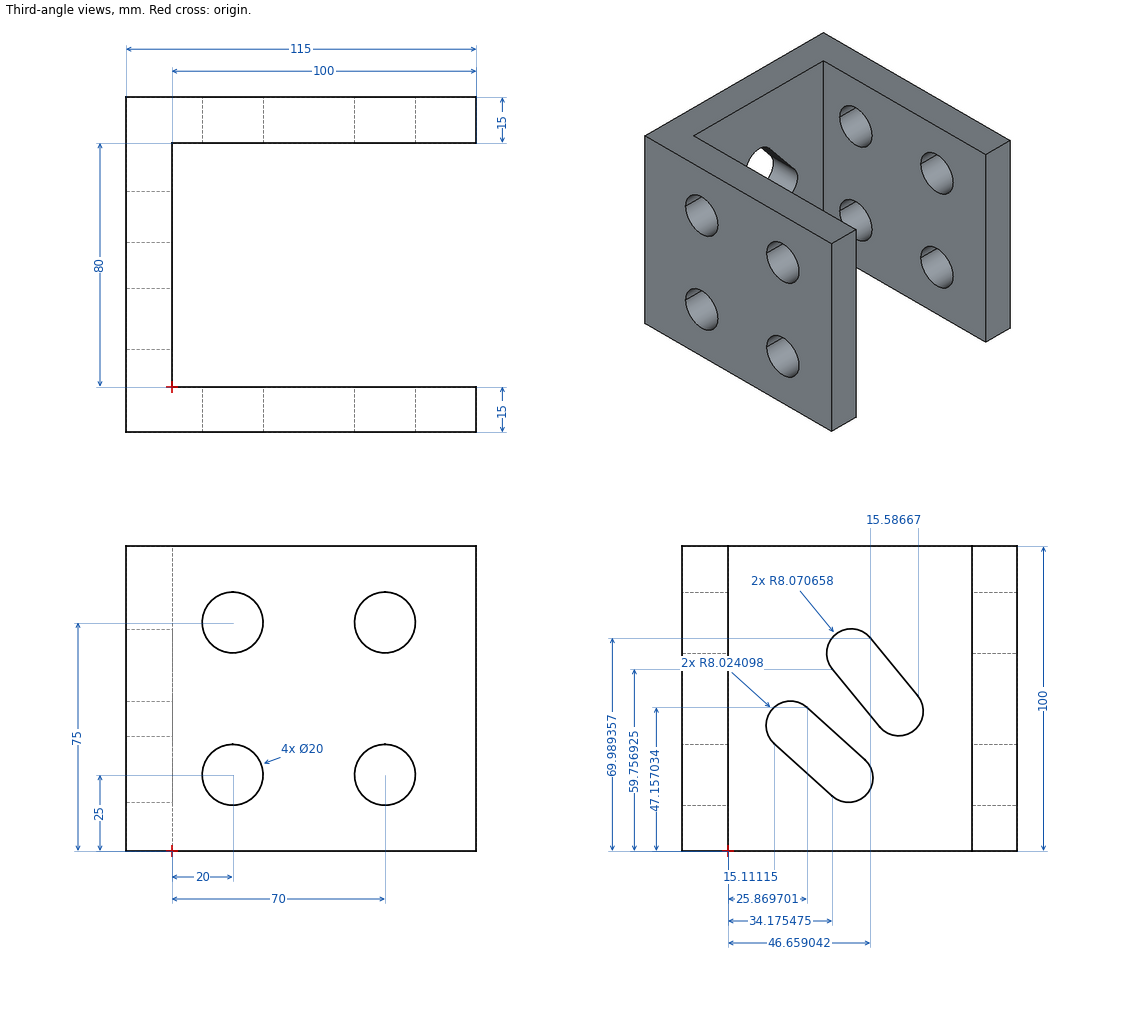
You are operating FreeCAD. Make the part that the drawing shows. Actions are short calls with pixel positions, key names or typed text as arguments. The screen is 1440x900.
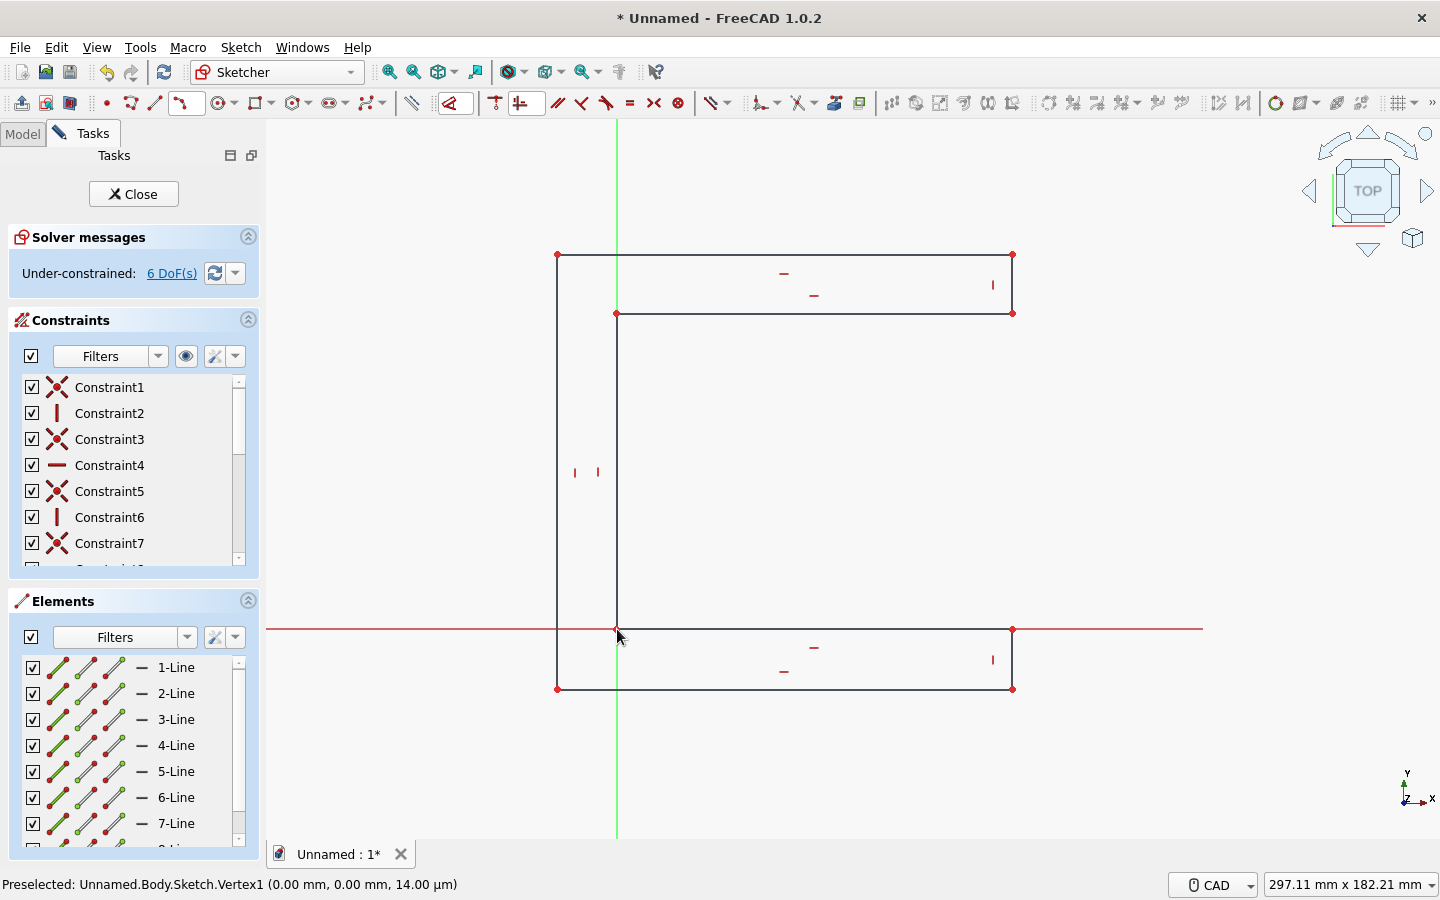
click(450, 104)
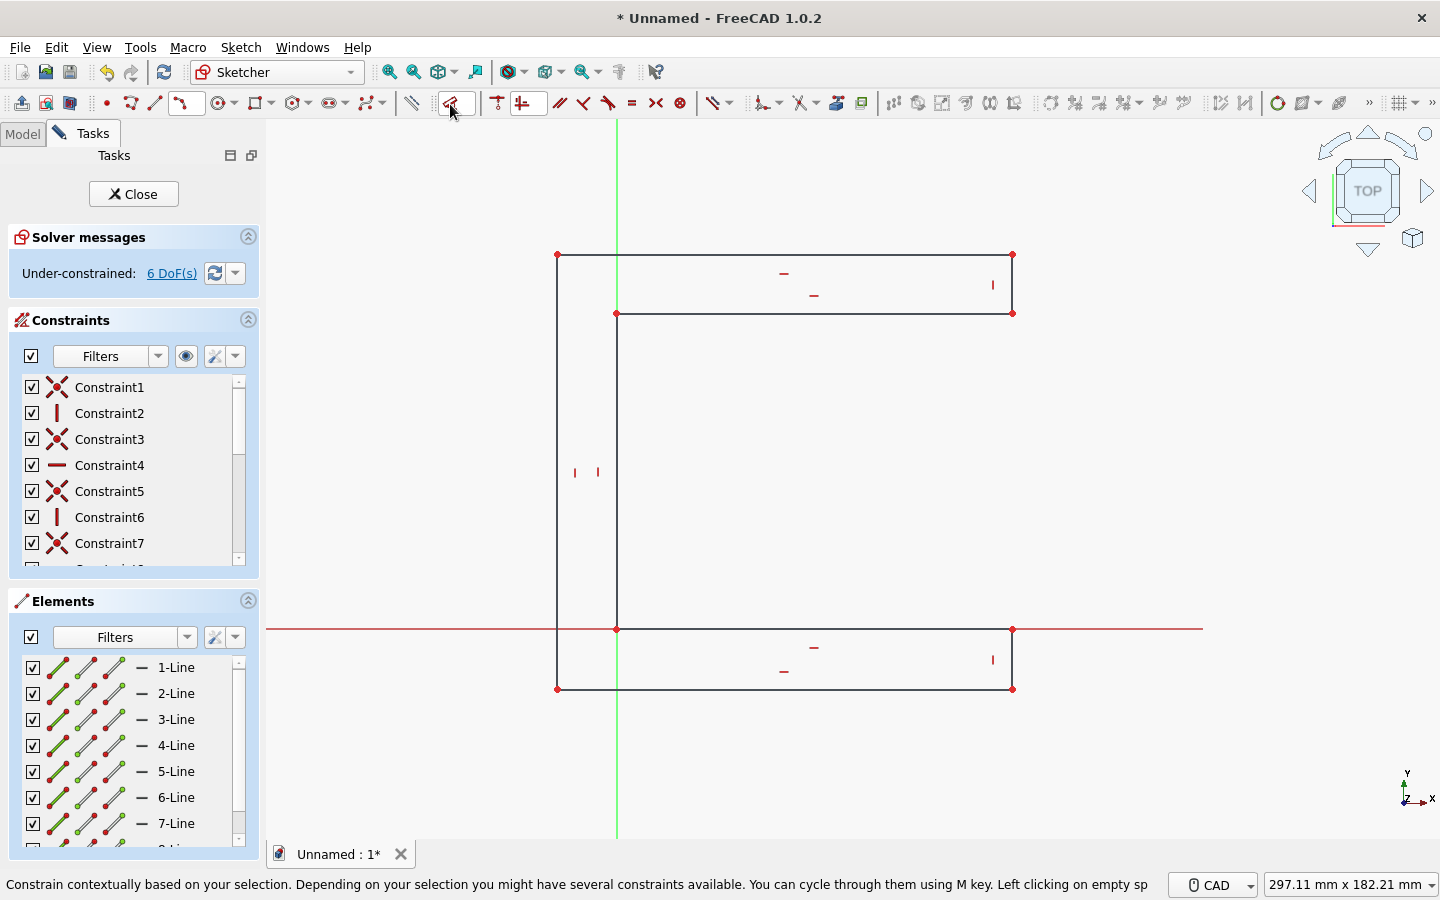
click(617, 535)
click(583, 472)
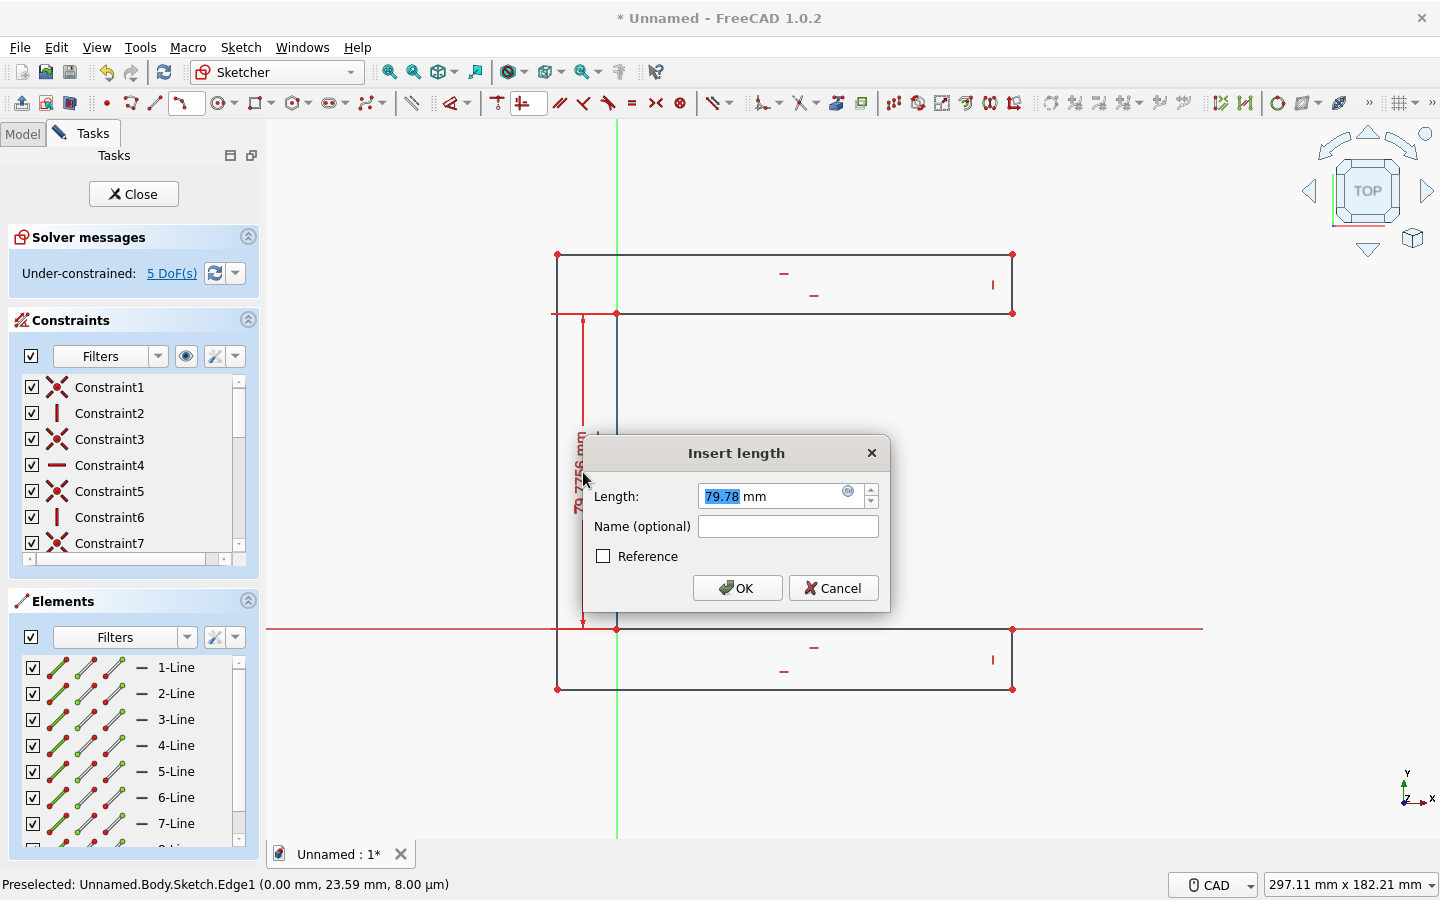
text(80)
key(Return)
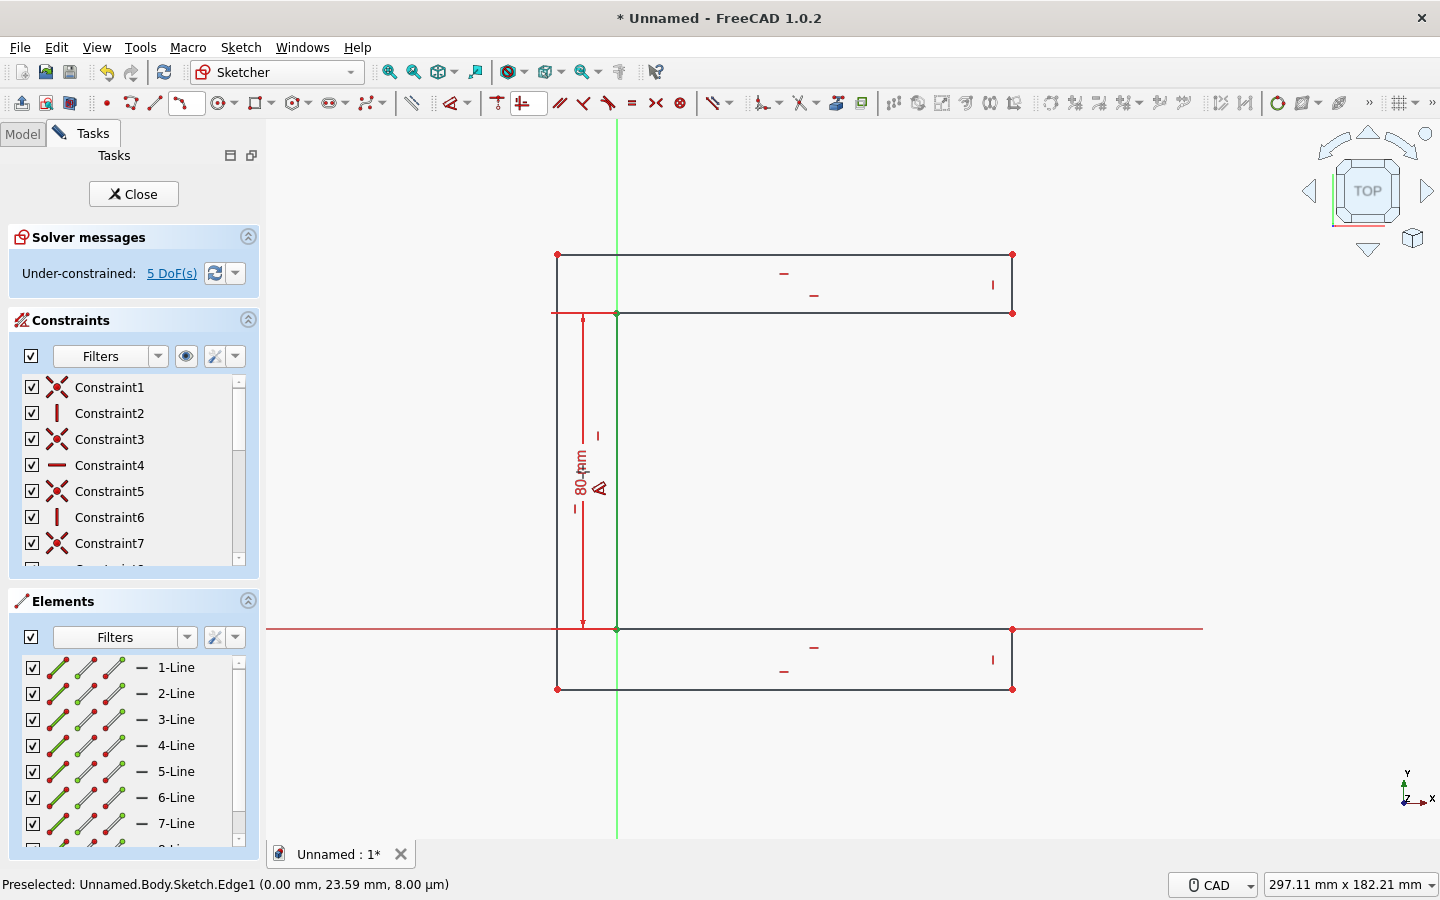
click(1012, 296)
click(1046, 284)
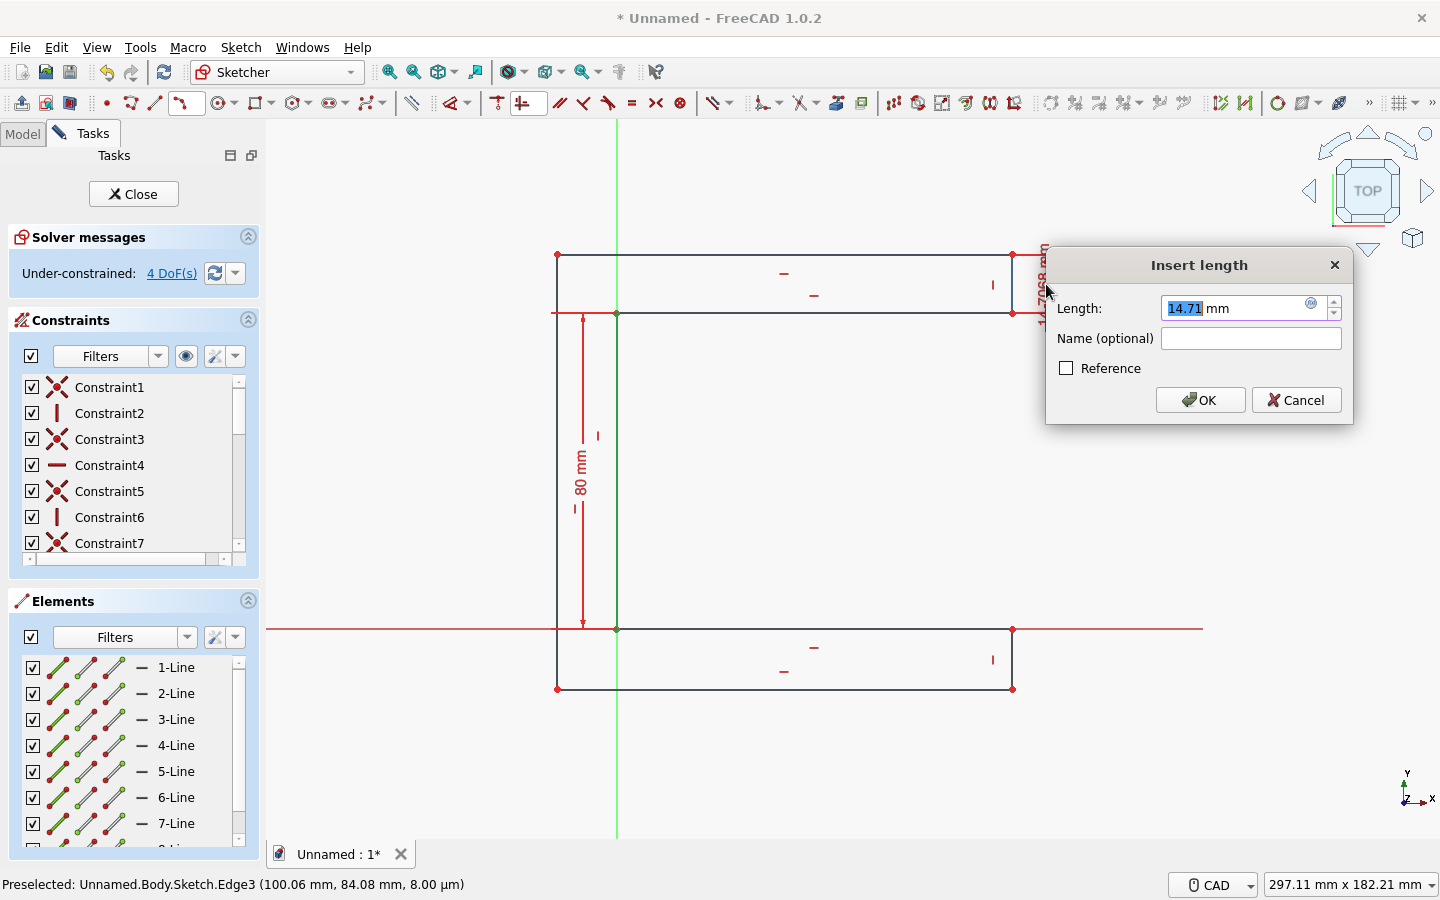
text(15)
key(Return)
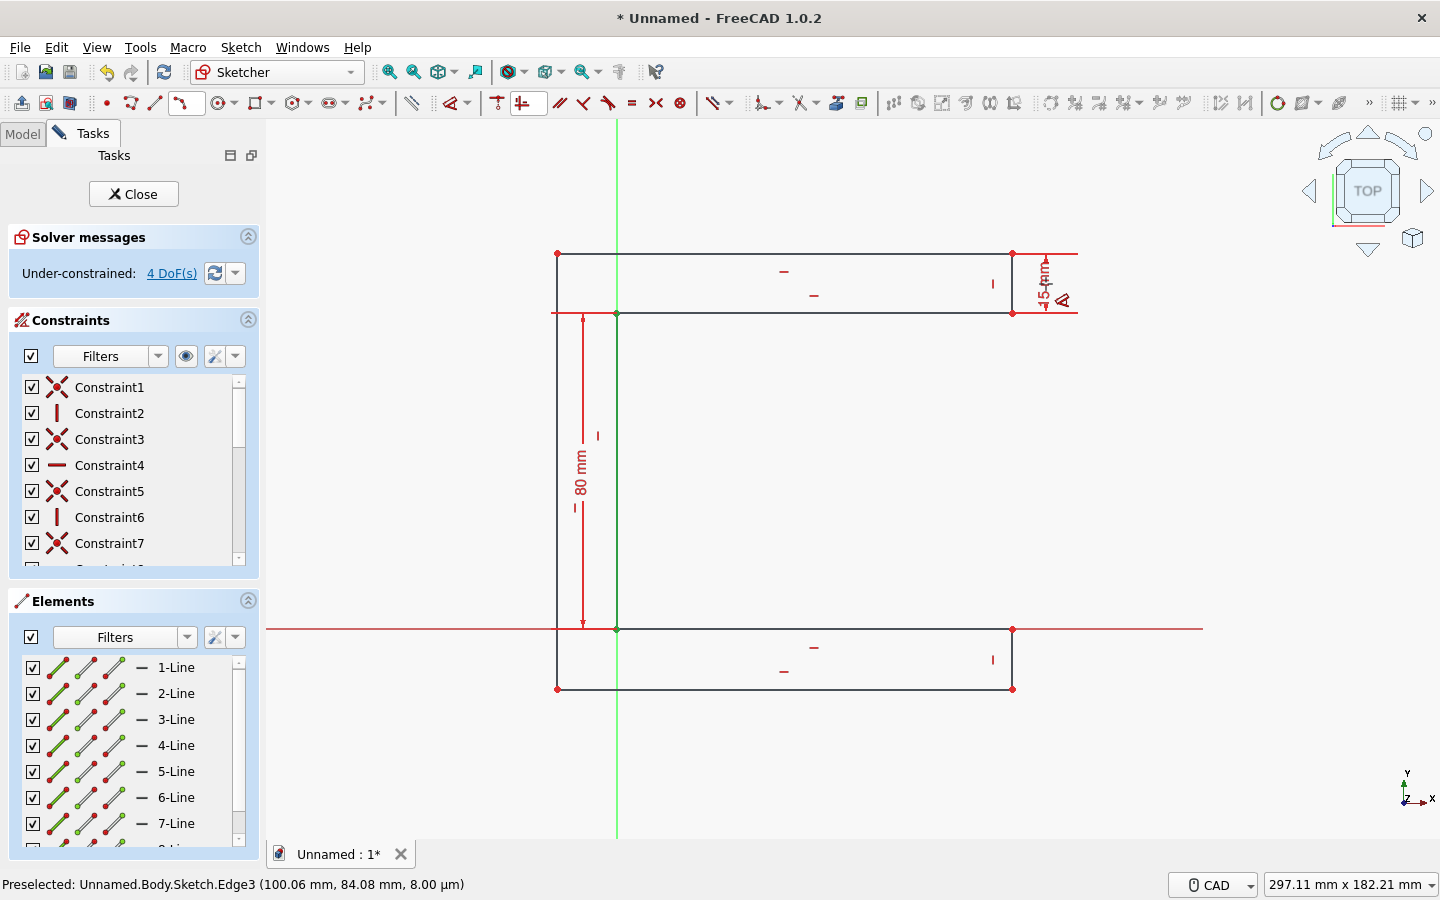
click(1012, 672)
click(1046, 660)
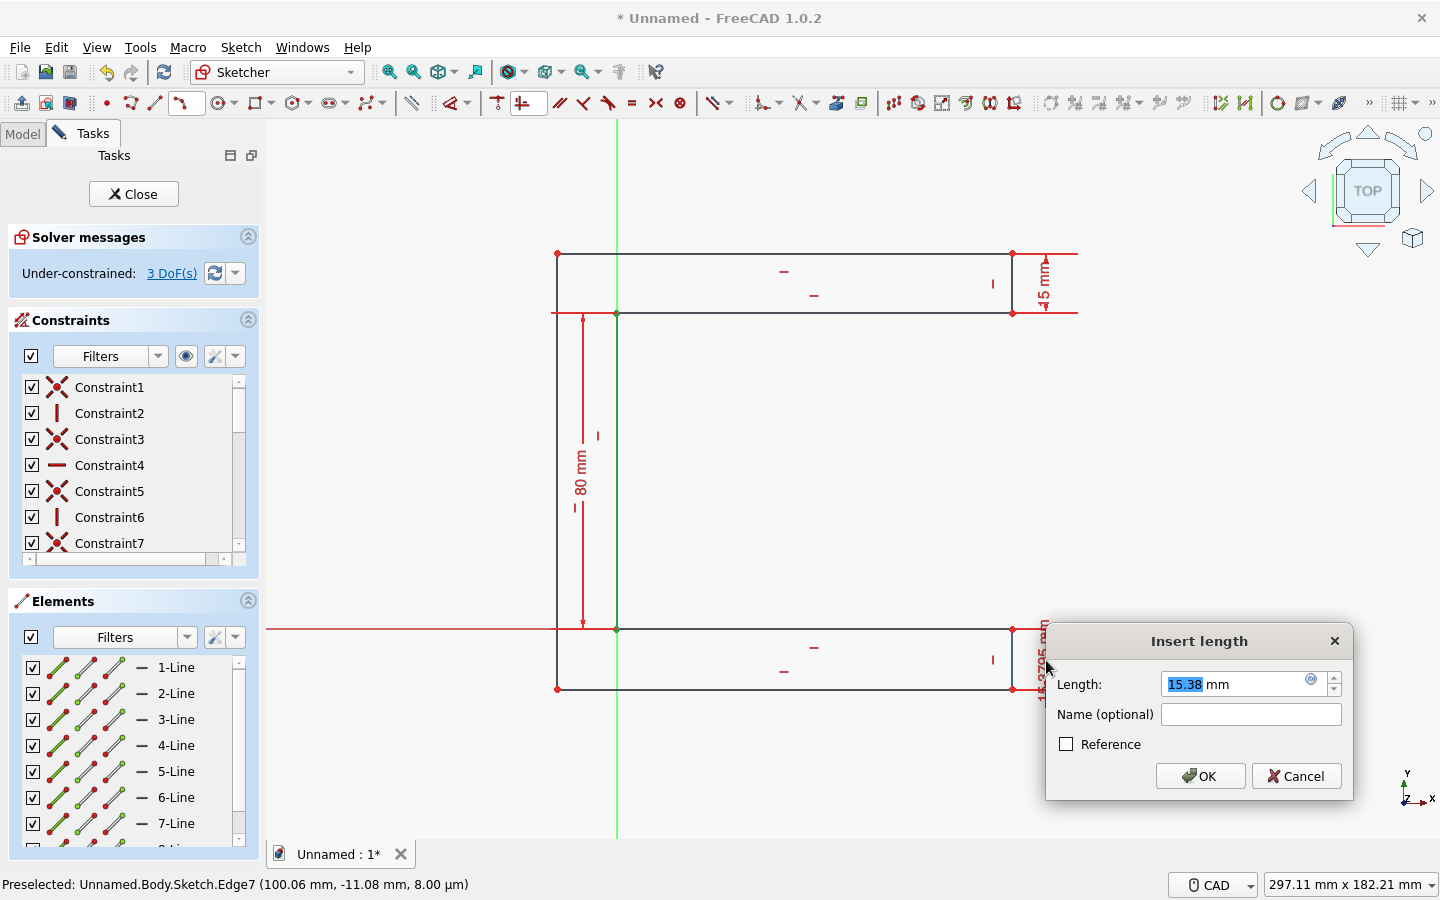
text(15)
key(Return)